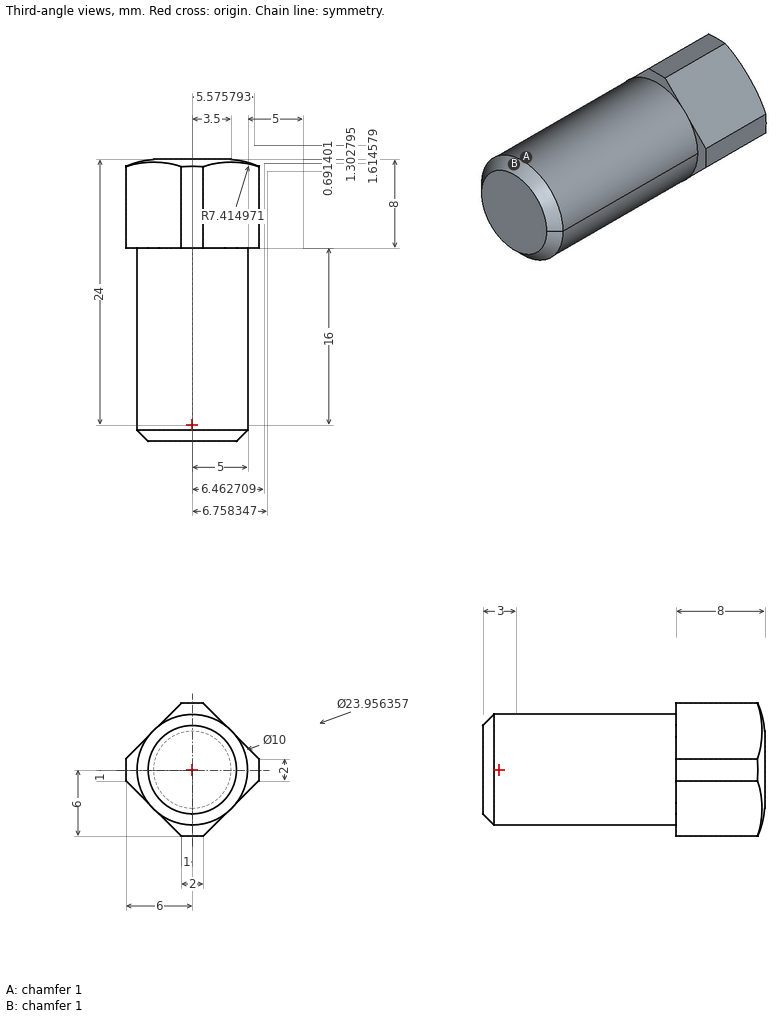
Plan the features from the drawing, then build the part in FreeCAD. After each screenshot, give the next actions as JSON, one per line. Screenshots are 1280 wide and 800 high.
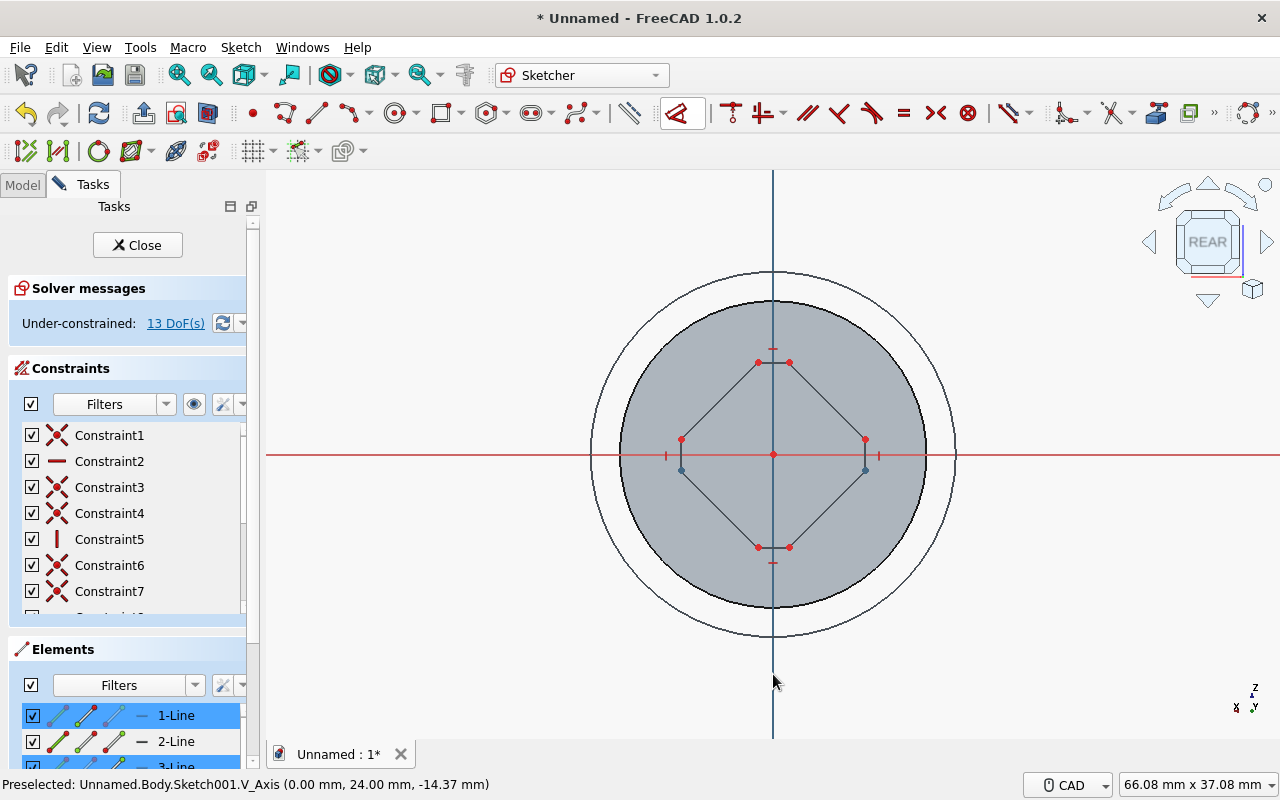
{"action": "left_click", "coordinate": [936, 114]}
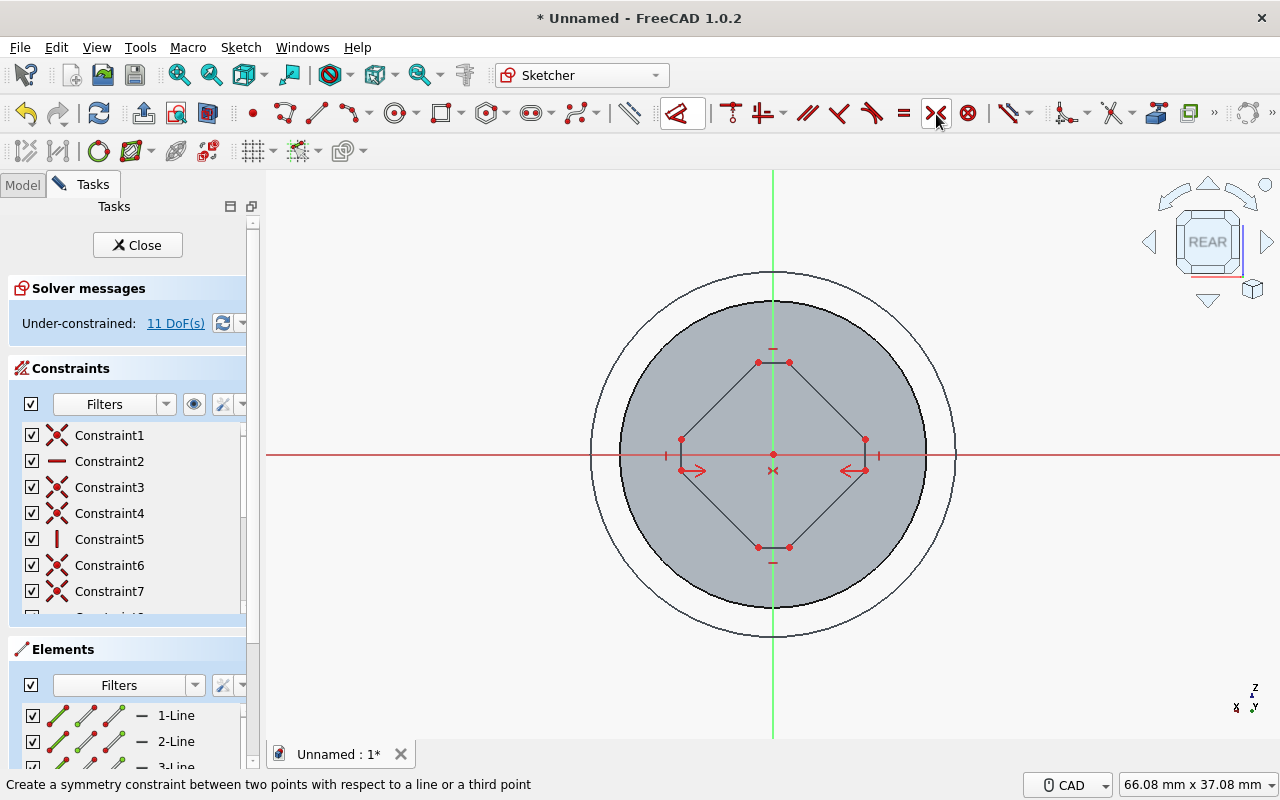
{"action": "left_click", "coordinate": [758, 548]}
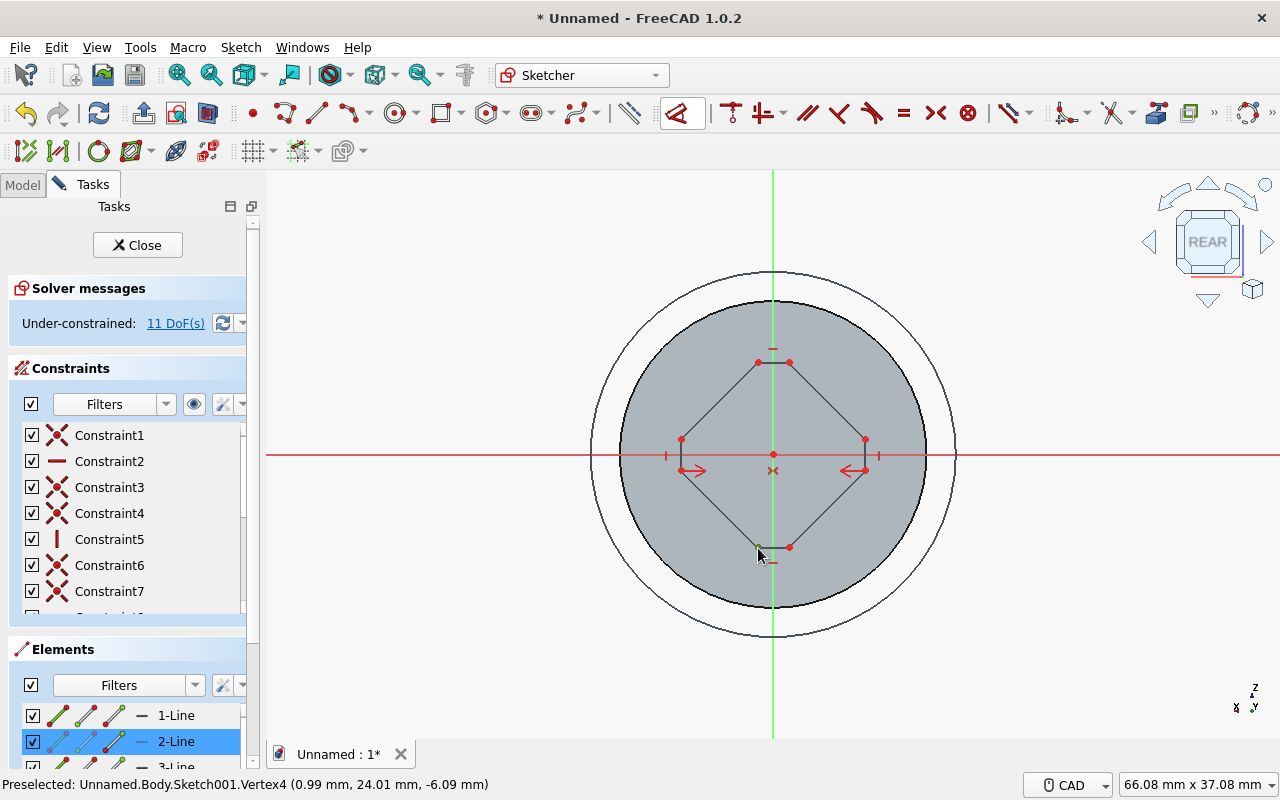
{"action": "left_click", "coordinate": [758, 363]}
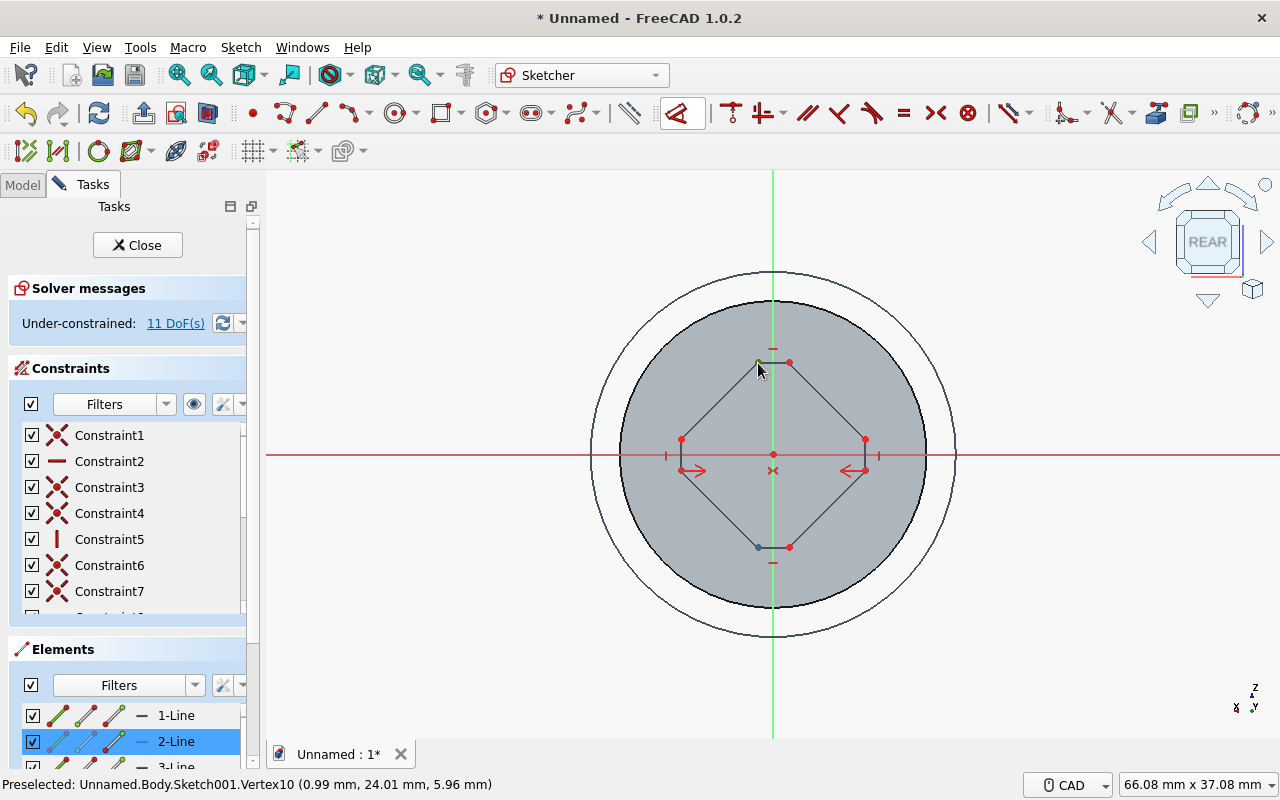
{"action": "left_click", "coordinate": [353, 455]}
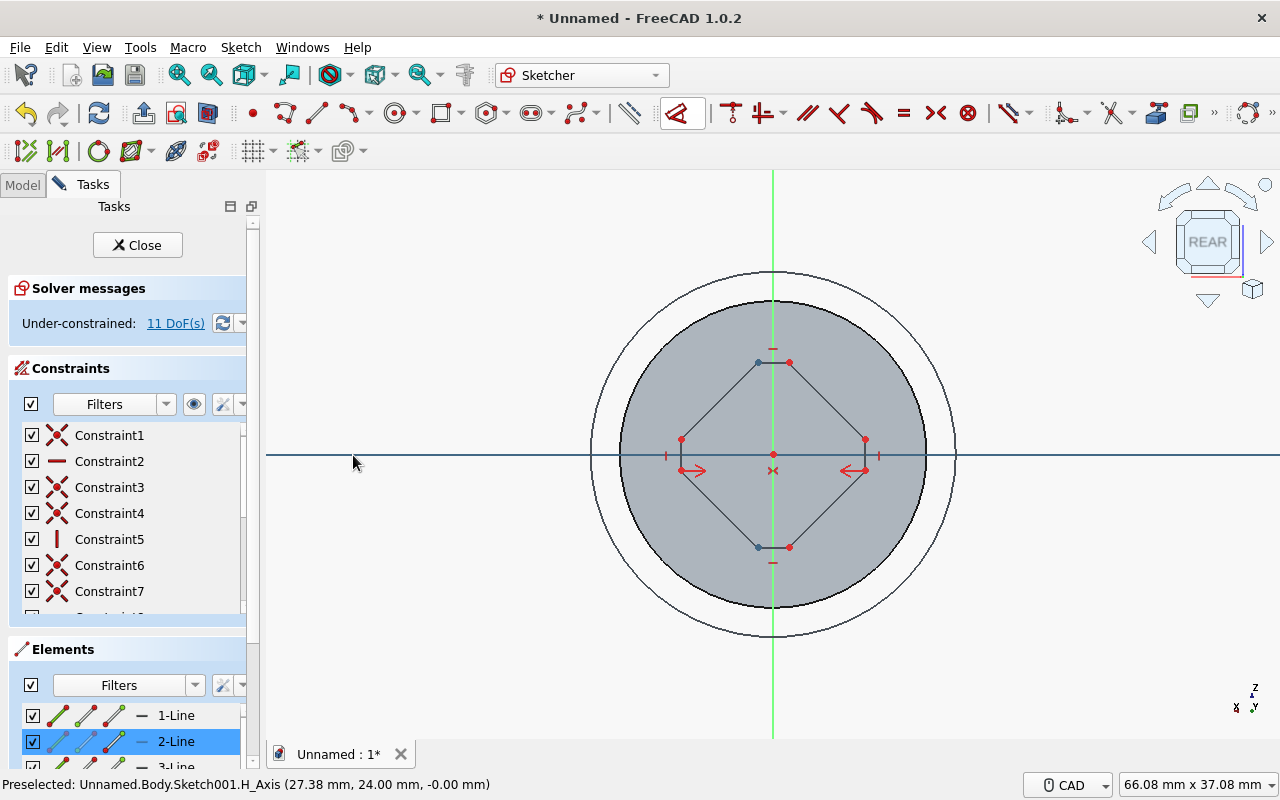
{"action": "left_click", "coordinate": [936, 114]}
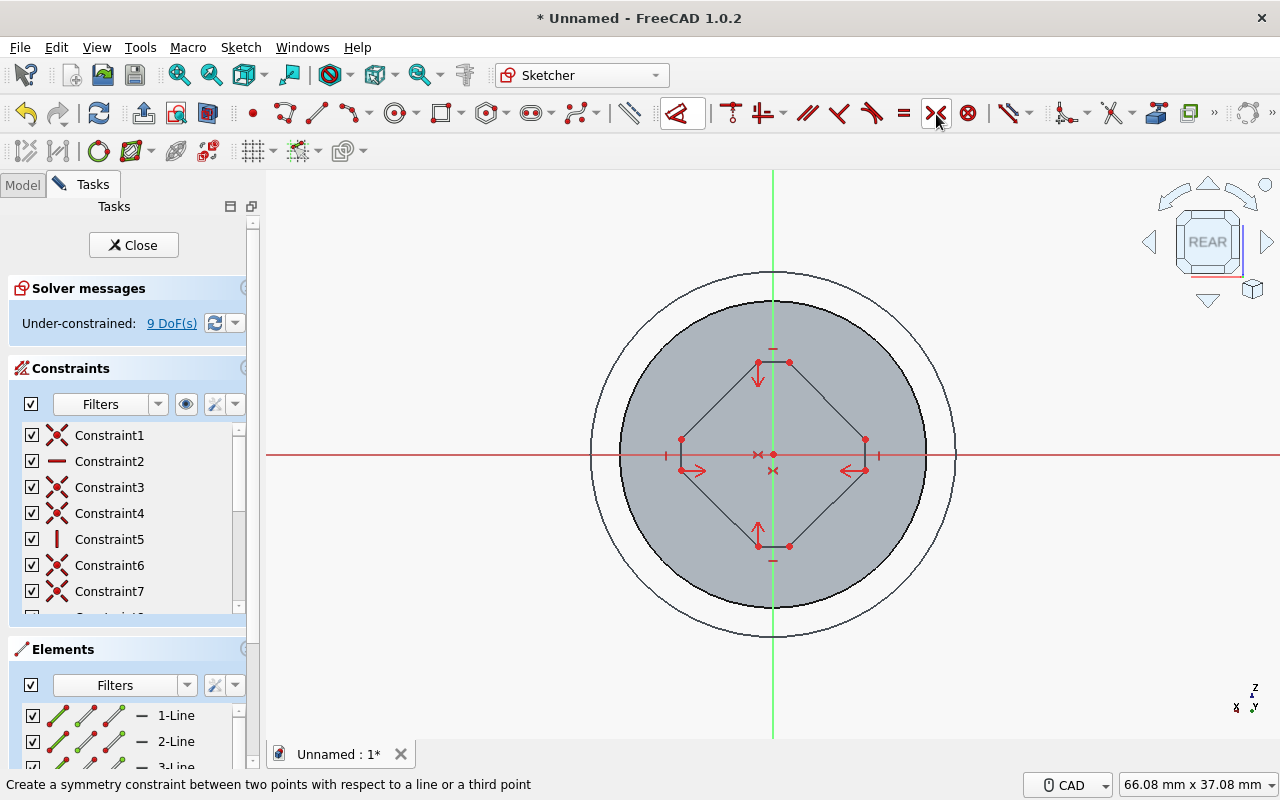
{"action": "left_click", "coordinate": [902, 325]}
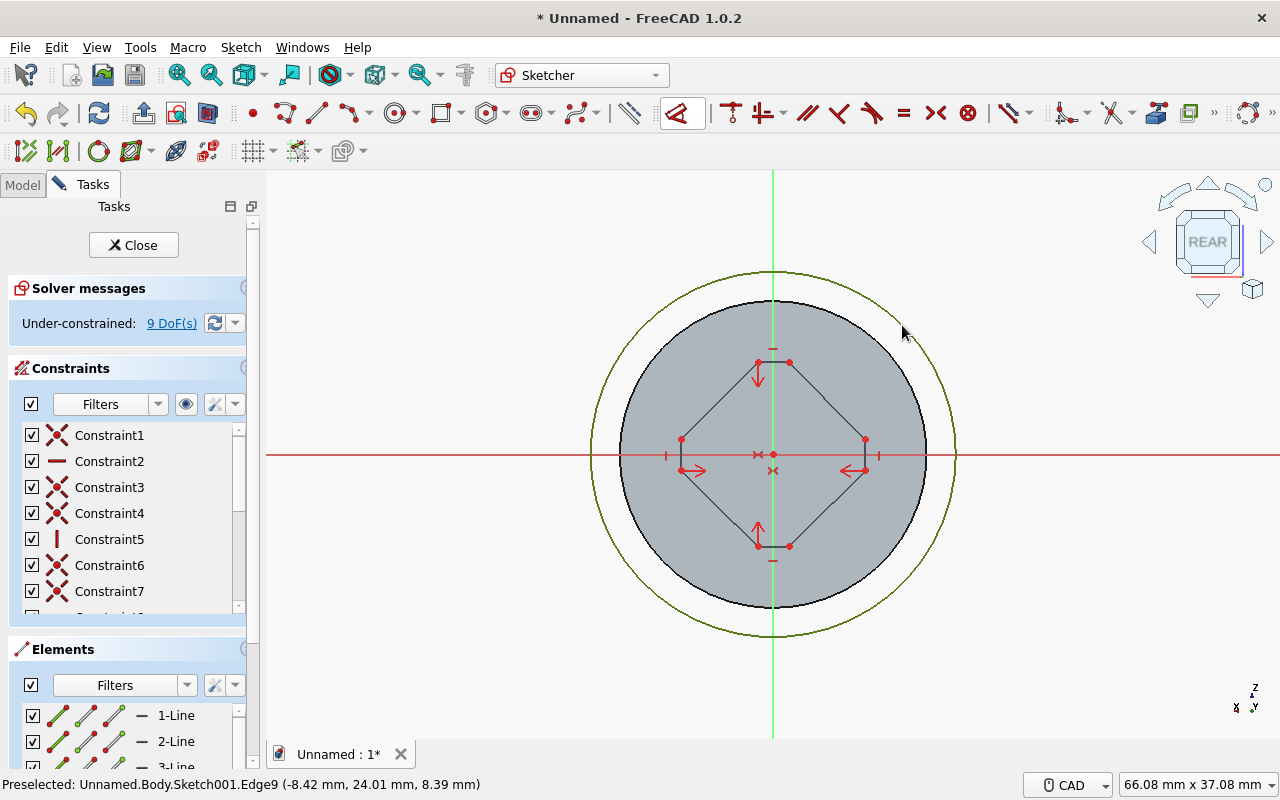
{"action": "left_click", "coordinate": [700, 114]}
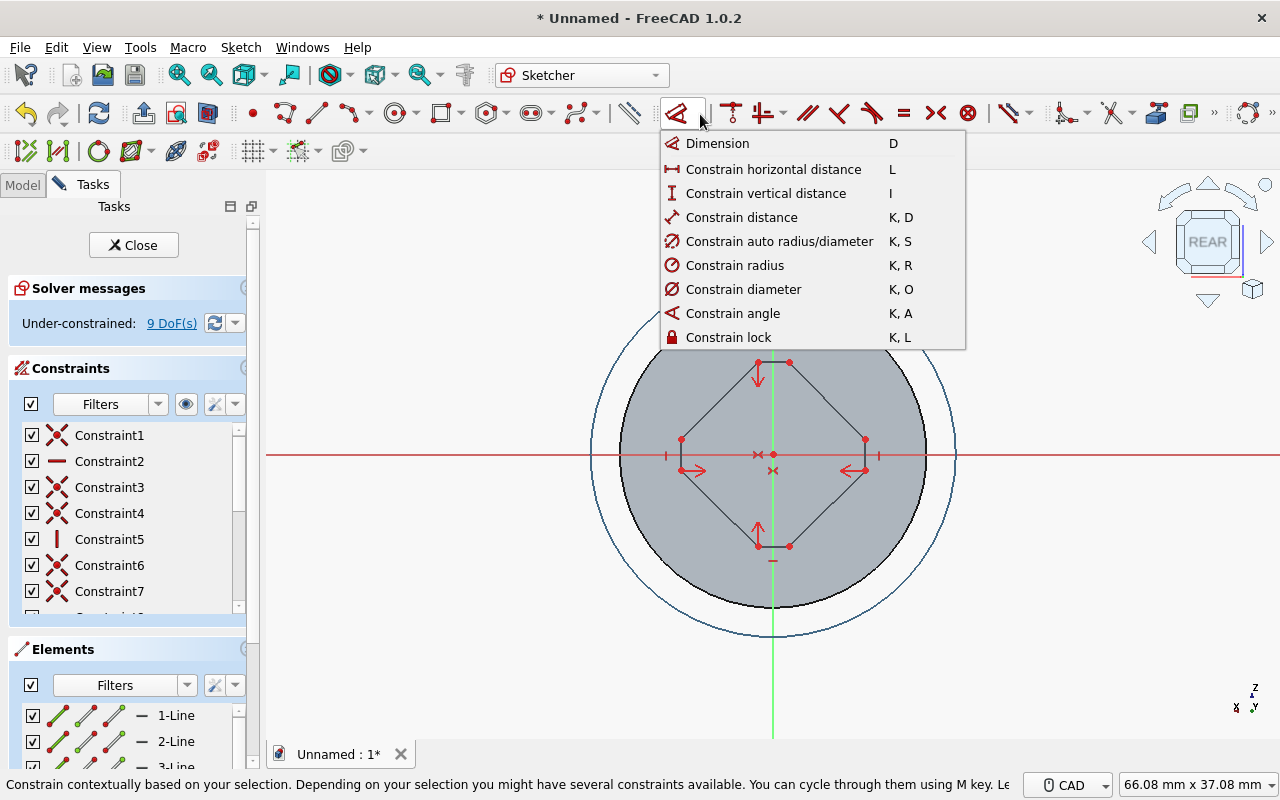
{"action": "left_click", "coordinate": [813, 289]}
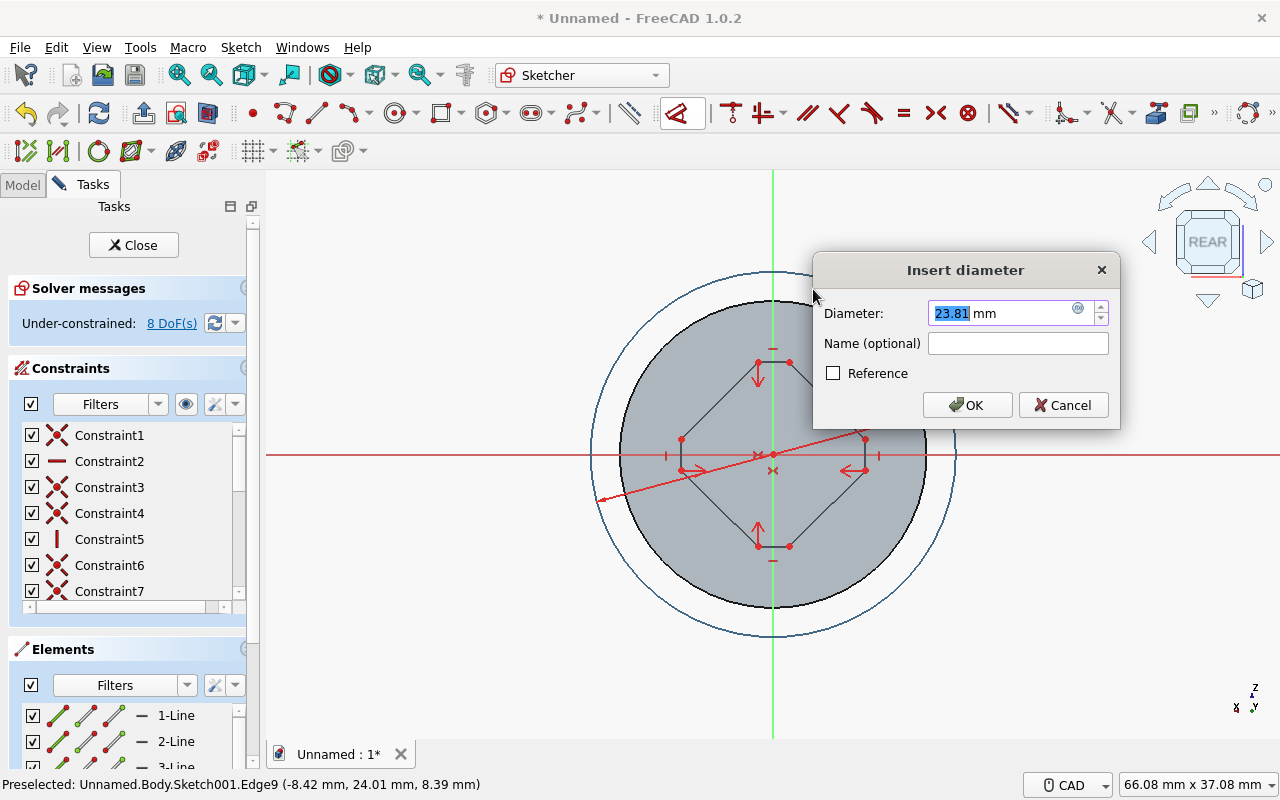
{"action": "type", "text": "23.956357"}
{"action": "key", "text": "Return"}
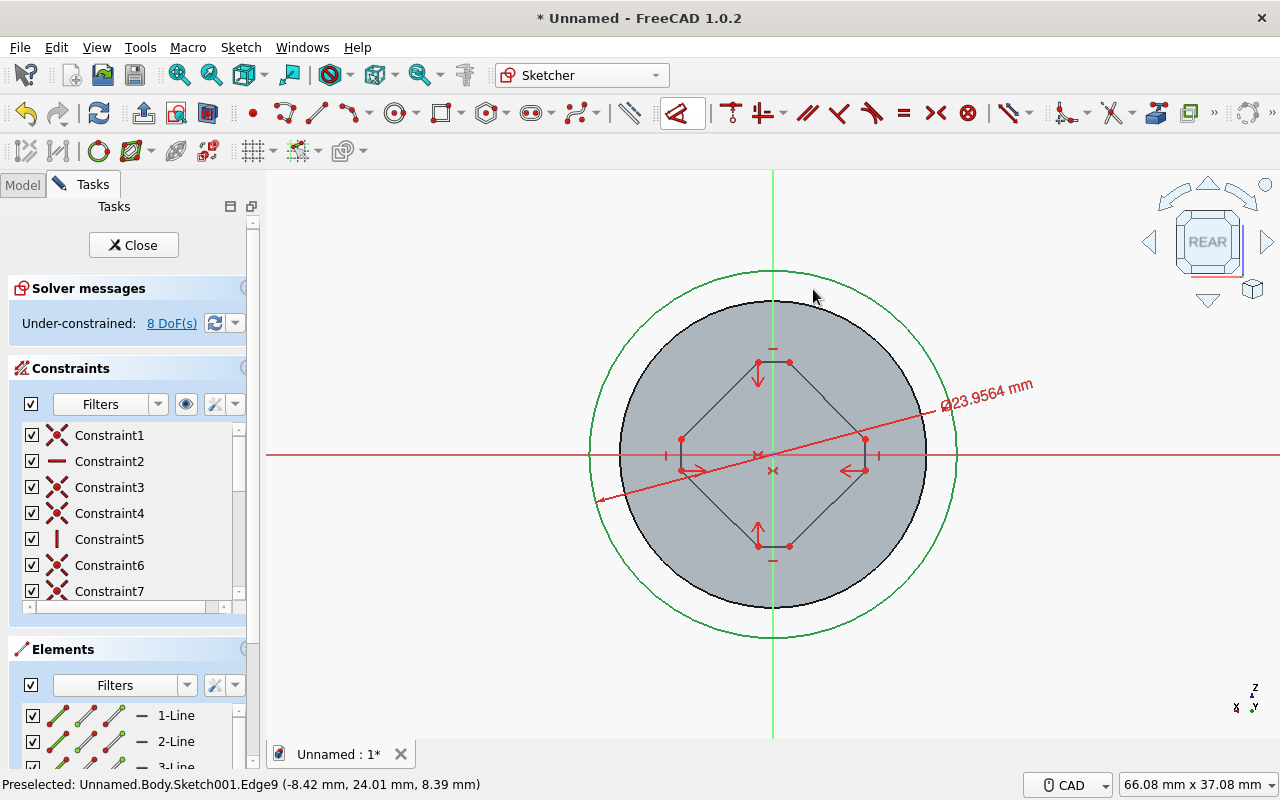
{"action": "scroll", "coordinate": [777, 547], "scroll_direction": "up", "scroll_amount": 2}